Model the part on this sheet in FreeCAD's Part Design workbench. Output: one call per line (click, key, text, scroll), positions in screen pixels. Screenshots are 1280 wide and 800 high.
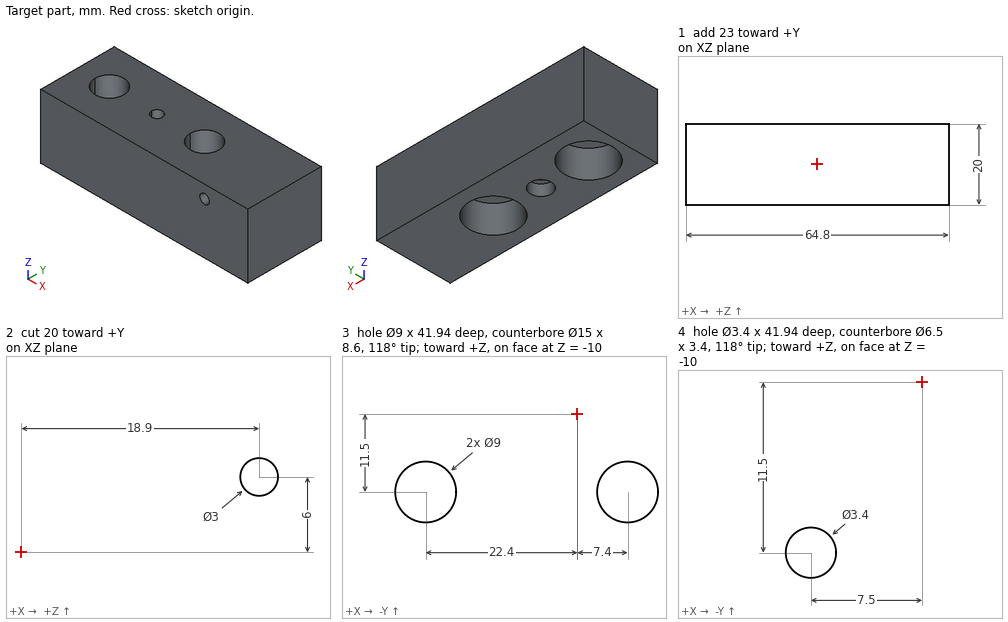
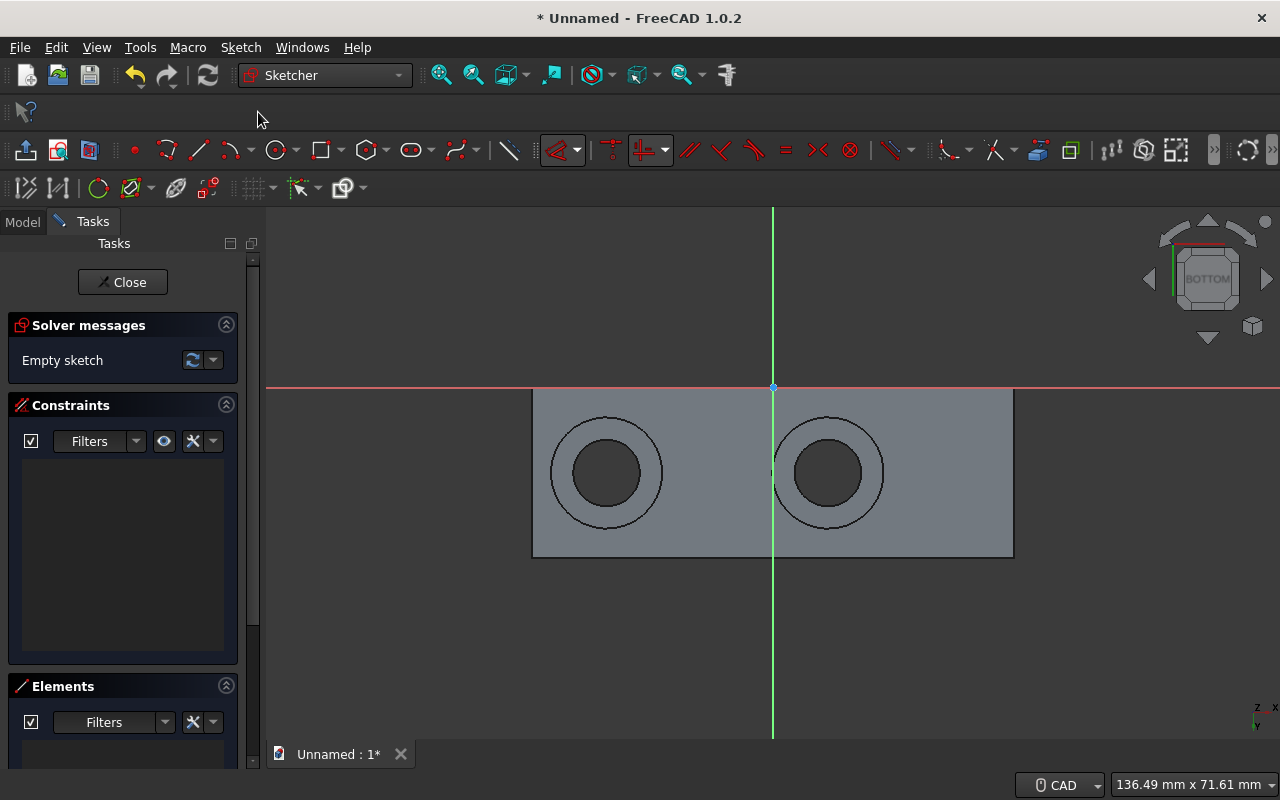
scroll(718, 473, up, 13)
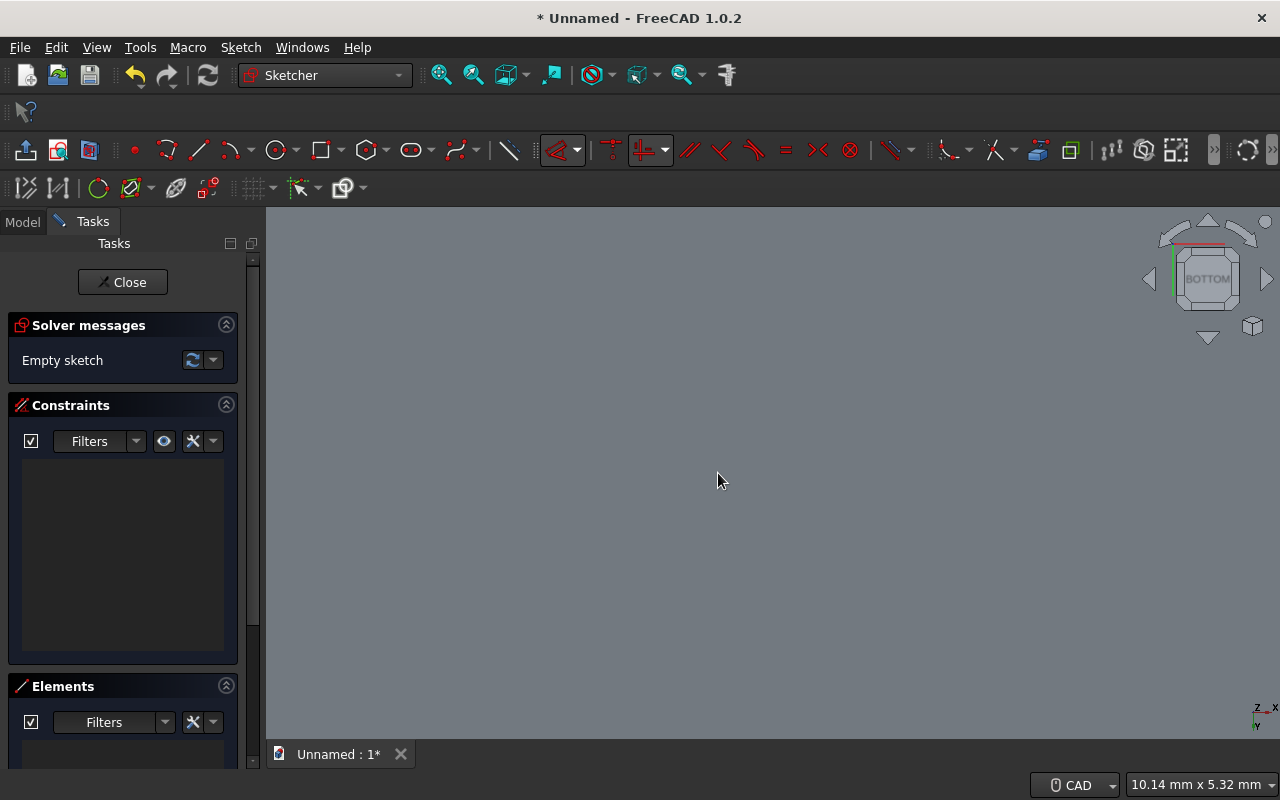
click(276, 150)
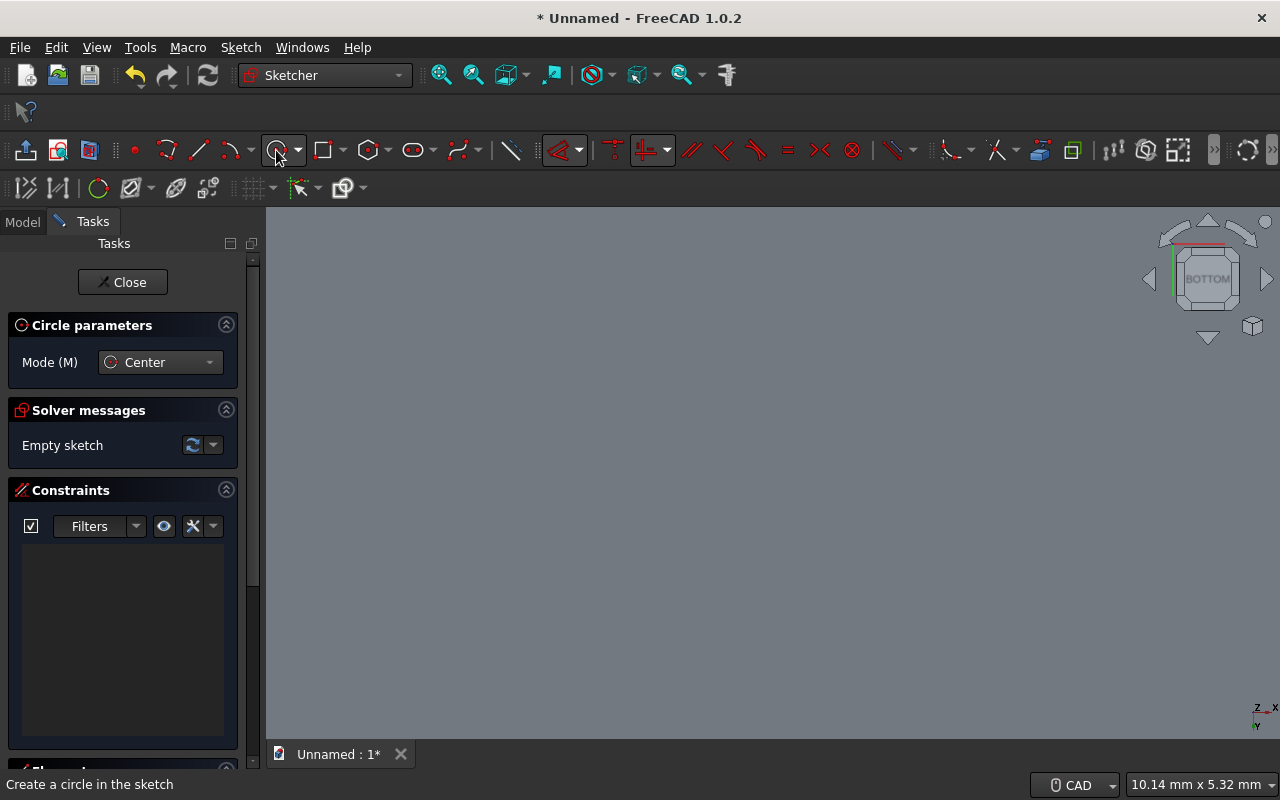
click(703, 467)
move(823, 347)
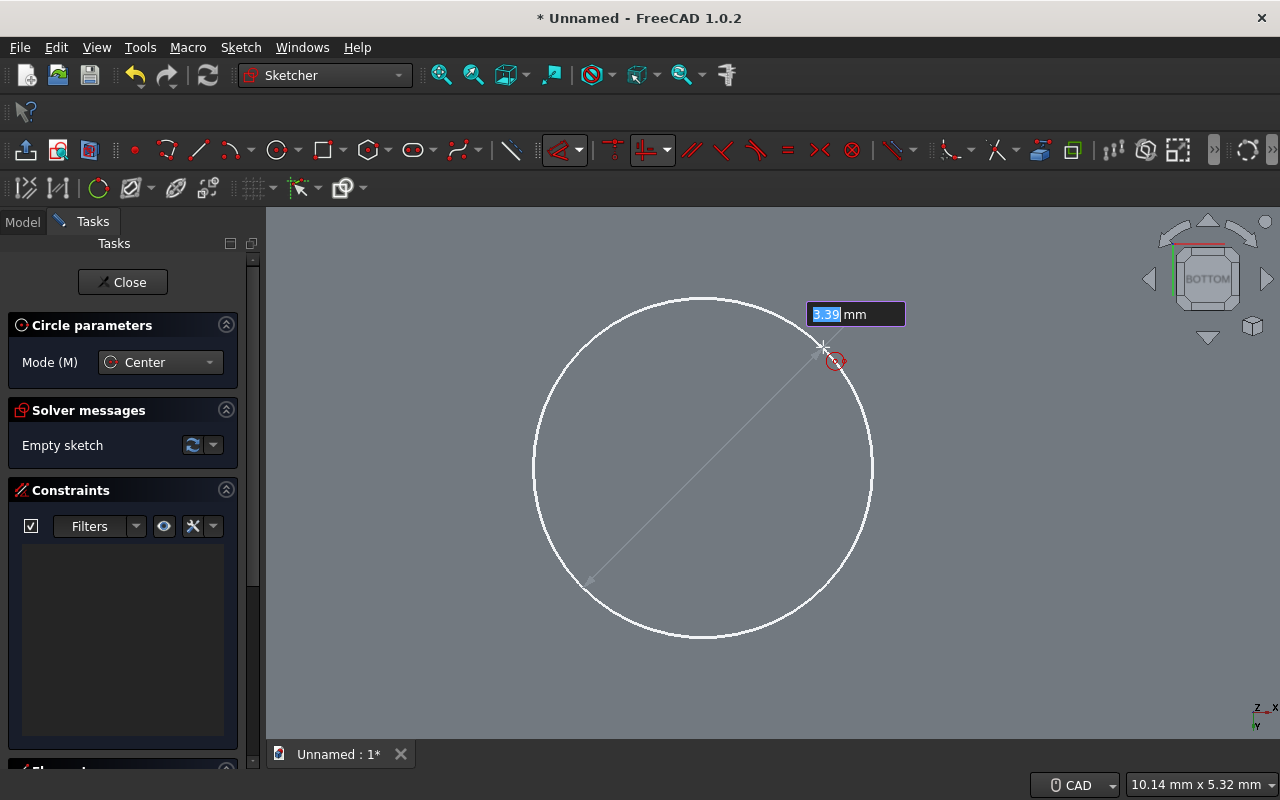
text(3.4)
key(Return)
key(Escape)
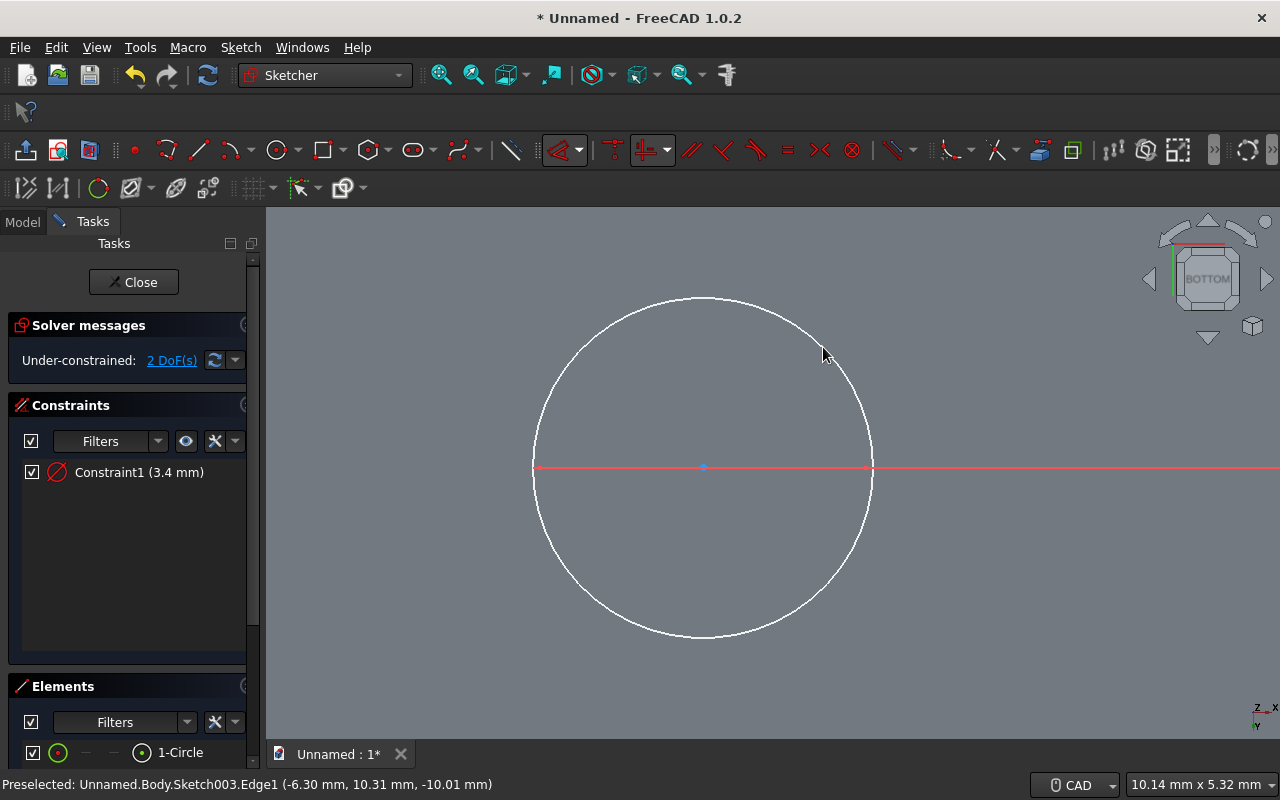
click(703, 468)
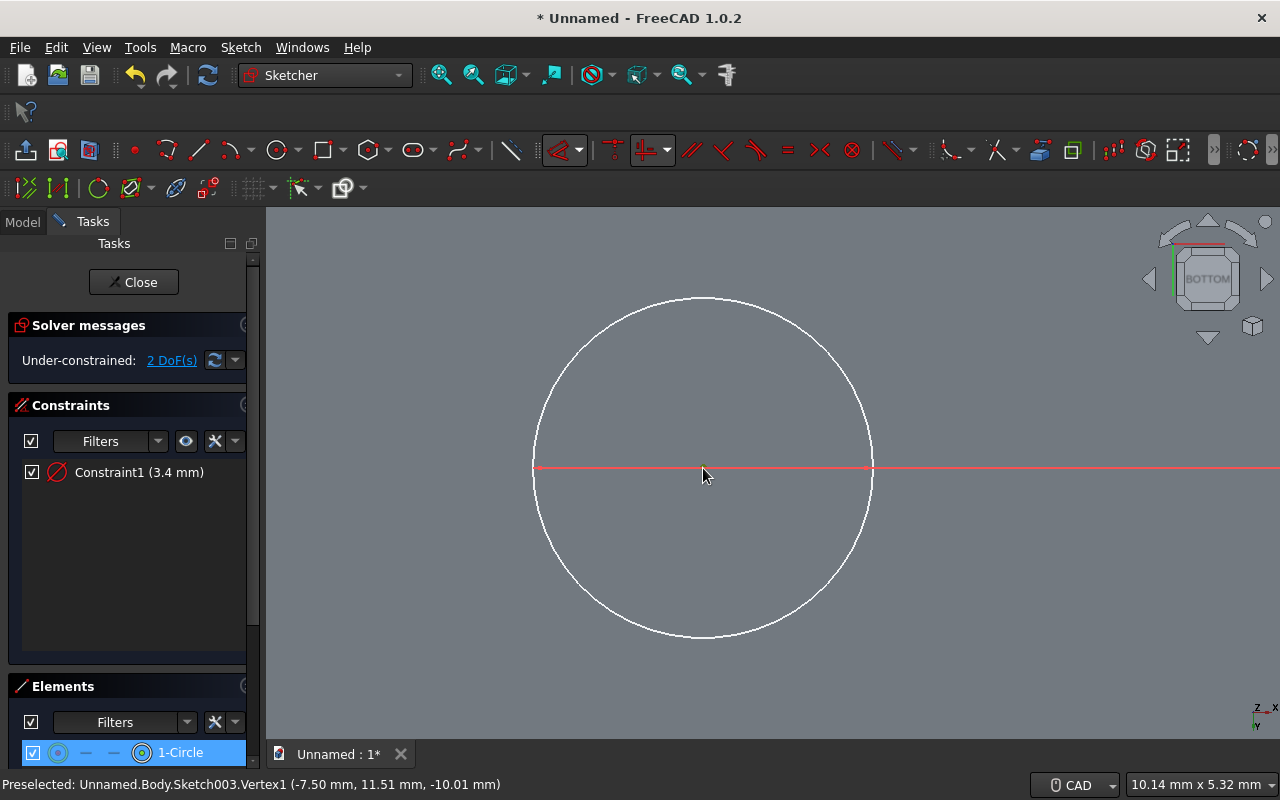
click(582, 150)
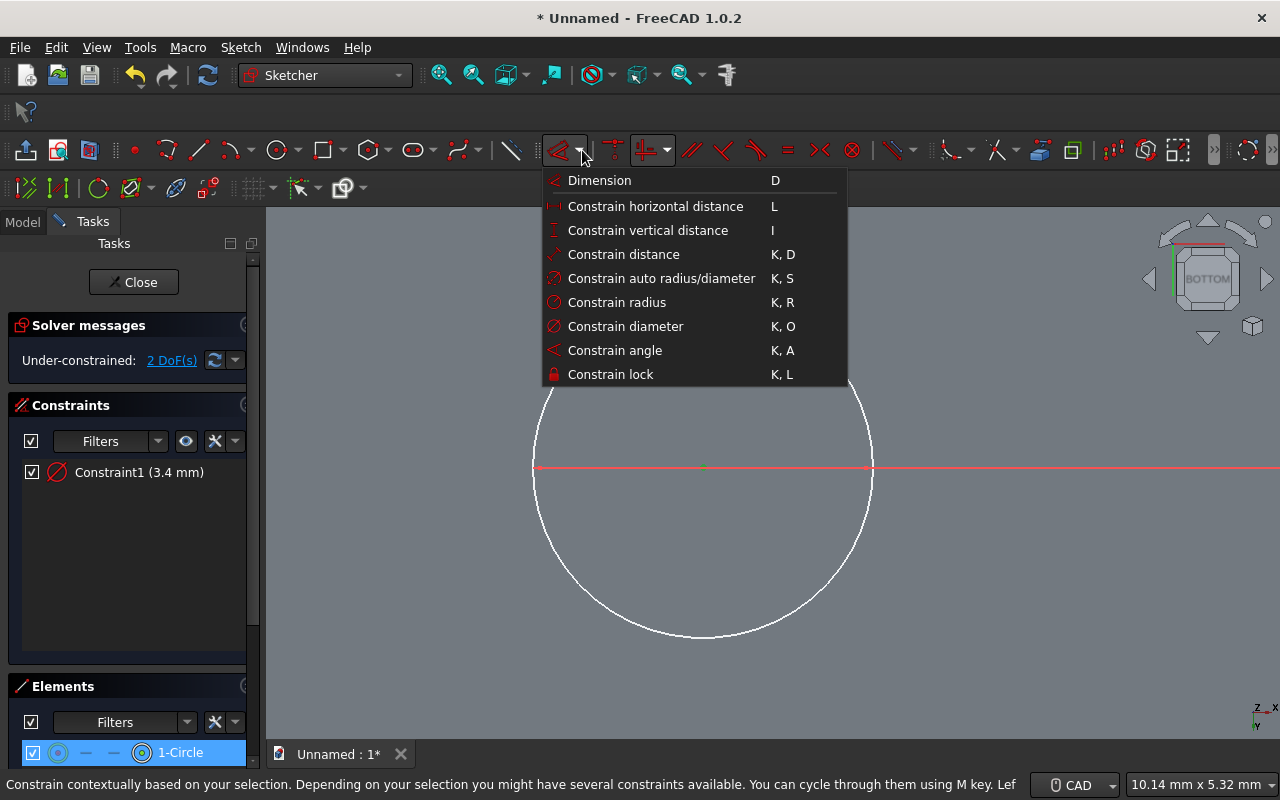
click(695, 206)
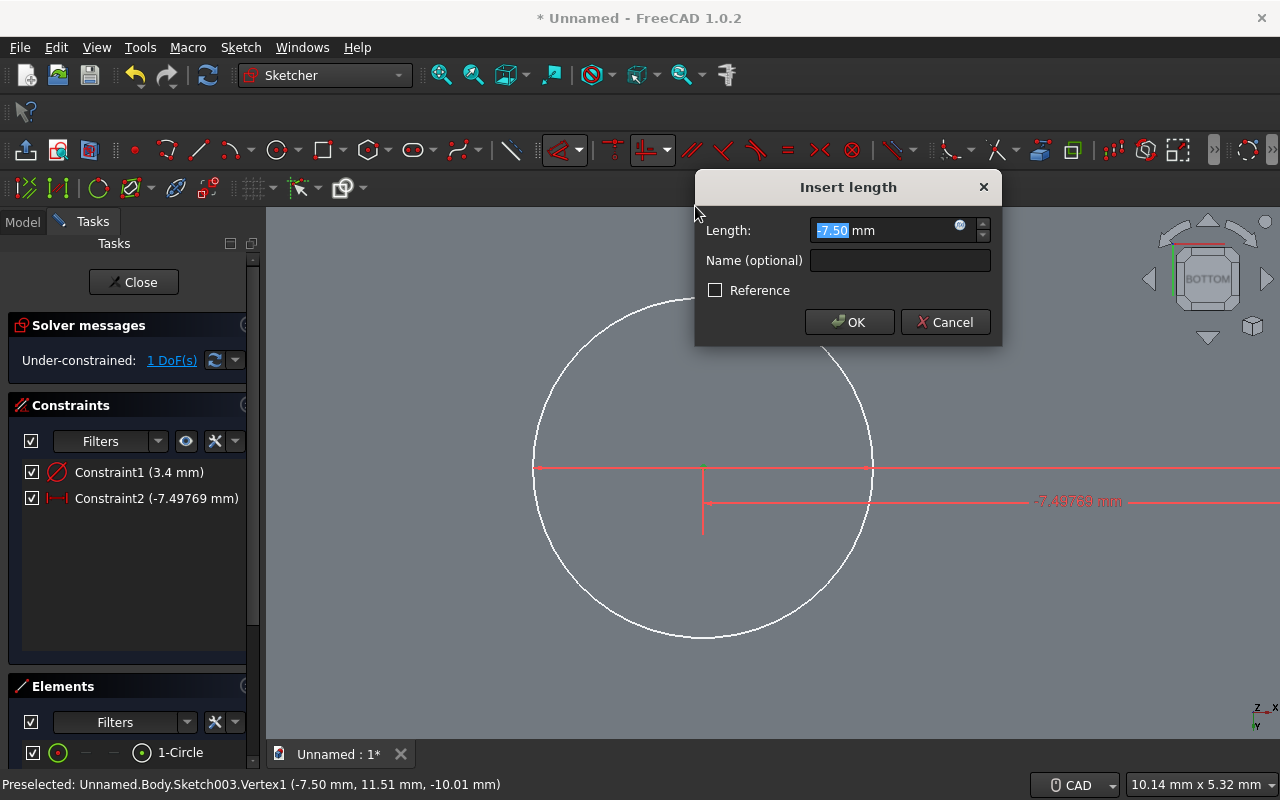
text(-7.5)
key(Return)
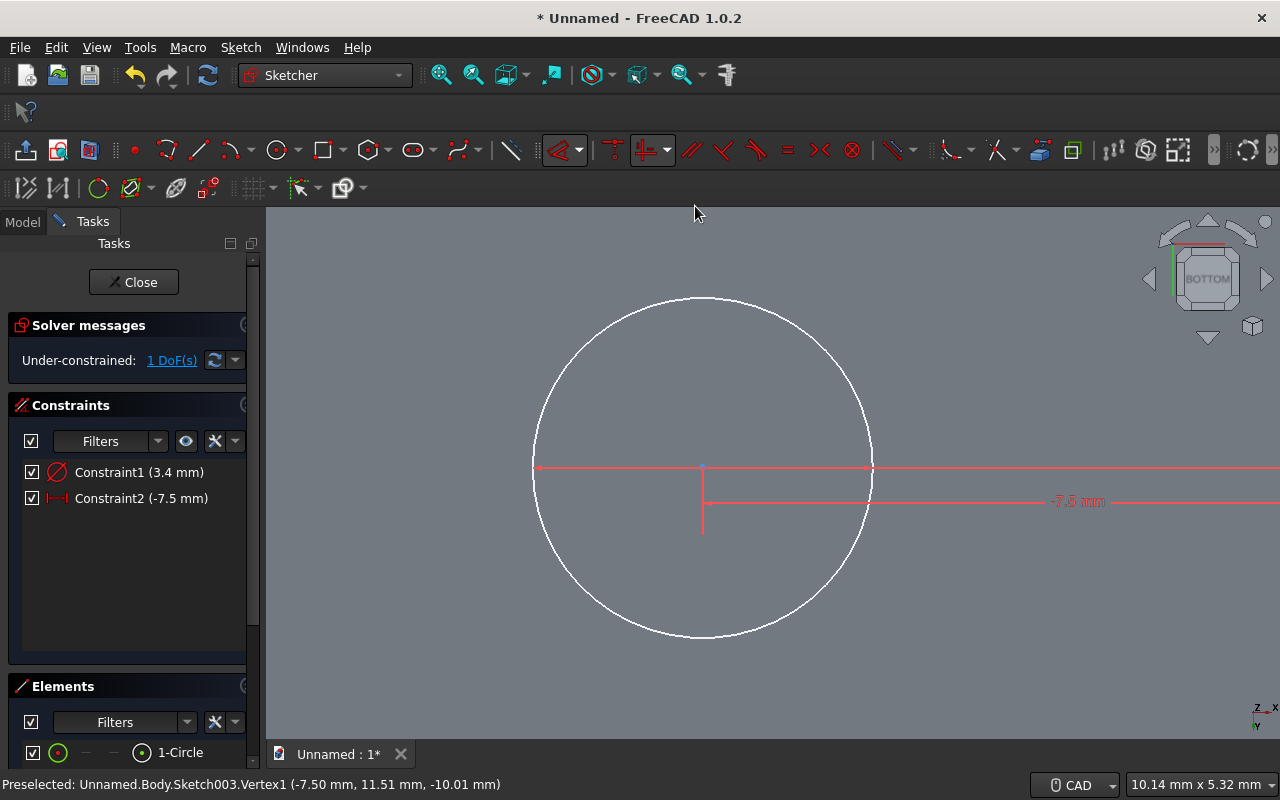
click(703, 468)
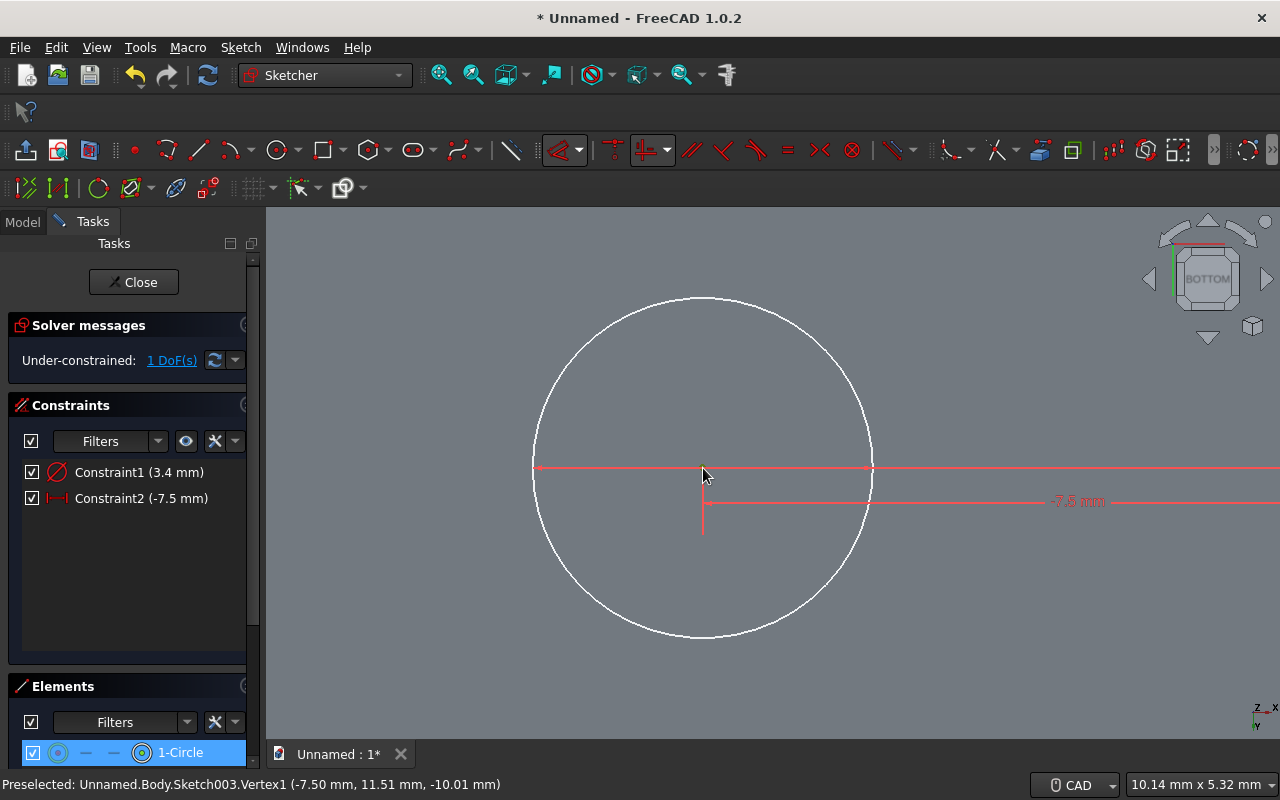
click(582, 150)